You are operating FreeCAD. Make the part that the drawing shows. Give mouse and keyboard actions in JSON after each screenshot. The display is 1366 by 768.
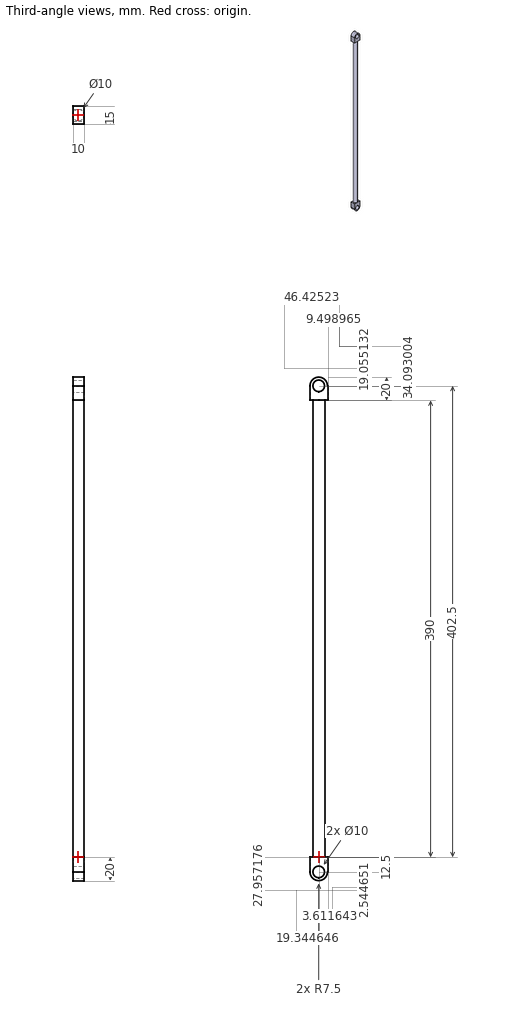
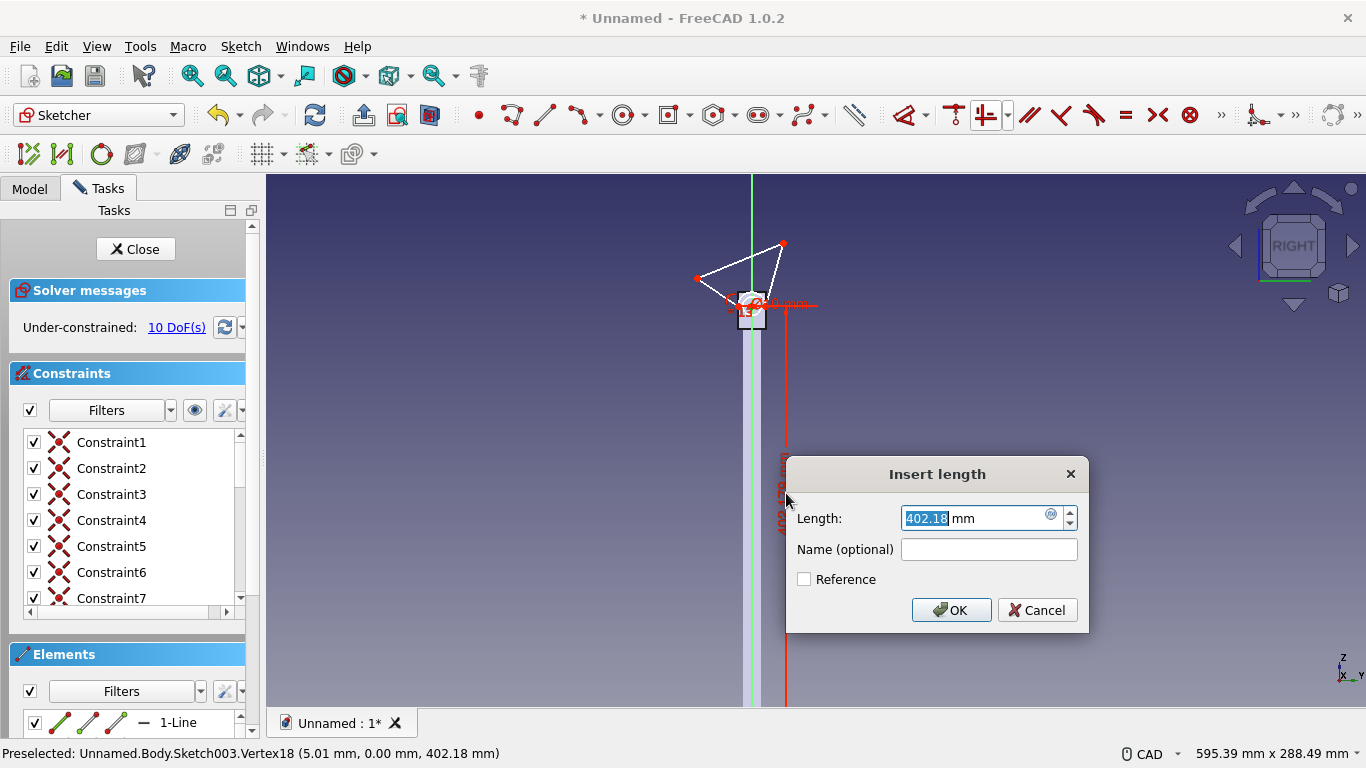
{"action": "type", "text": "402.5"}
{"action": "key", "text": "Return"}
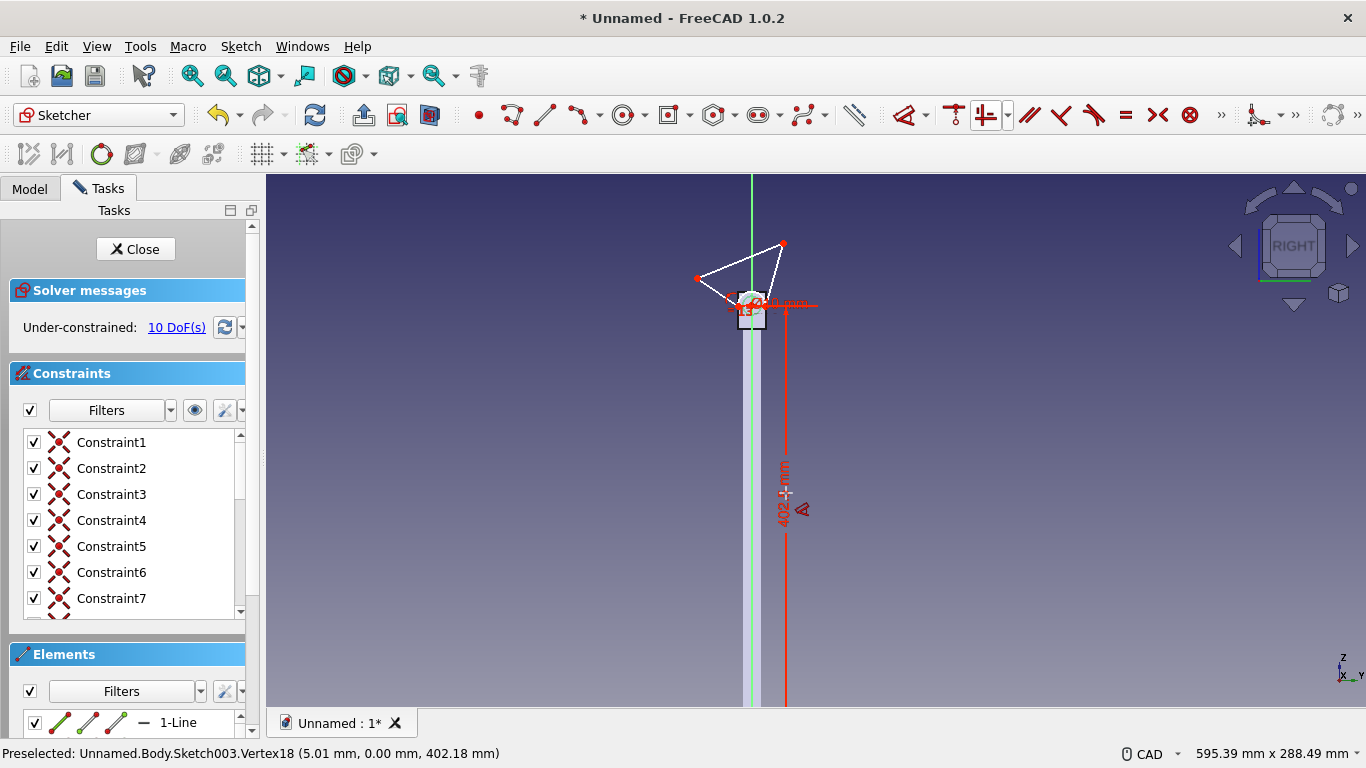
{"action": "left_click", "coordinate": [766, 306]}
{"action": "left_click", "coordinate": [800, 407]}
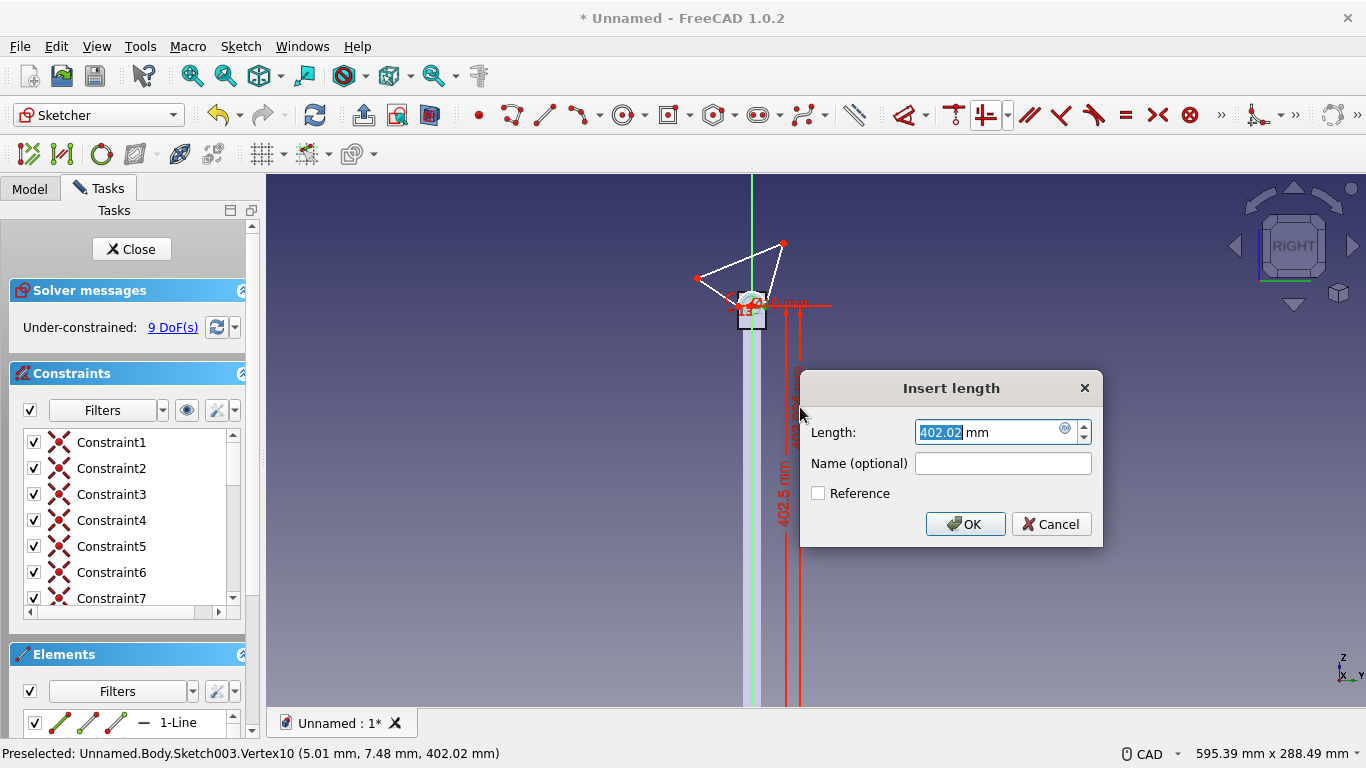
{"action": "type", "text": "402.5"}
{"action": "key", "text": "Return"}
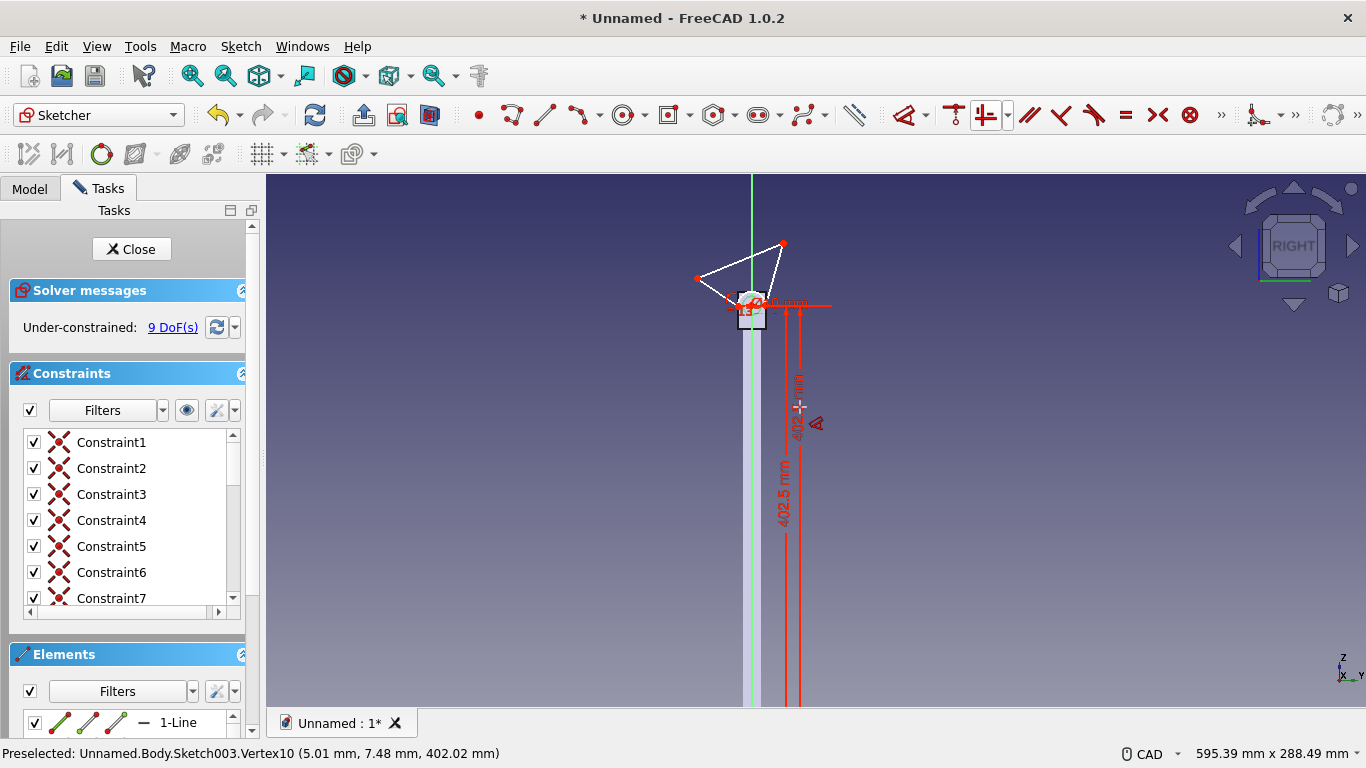
{"action": "left_click", "coordinate": [738, 306]}
{"action": "left_click", "coordinate": [786, 578]}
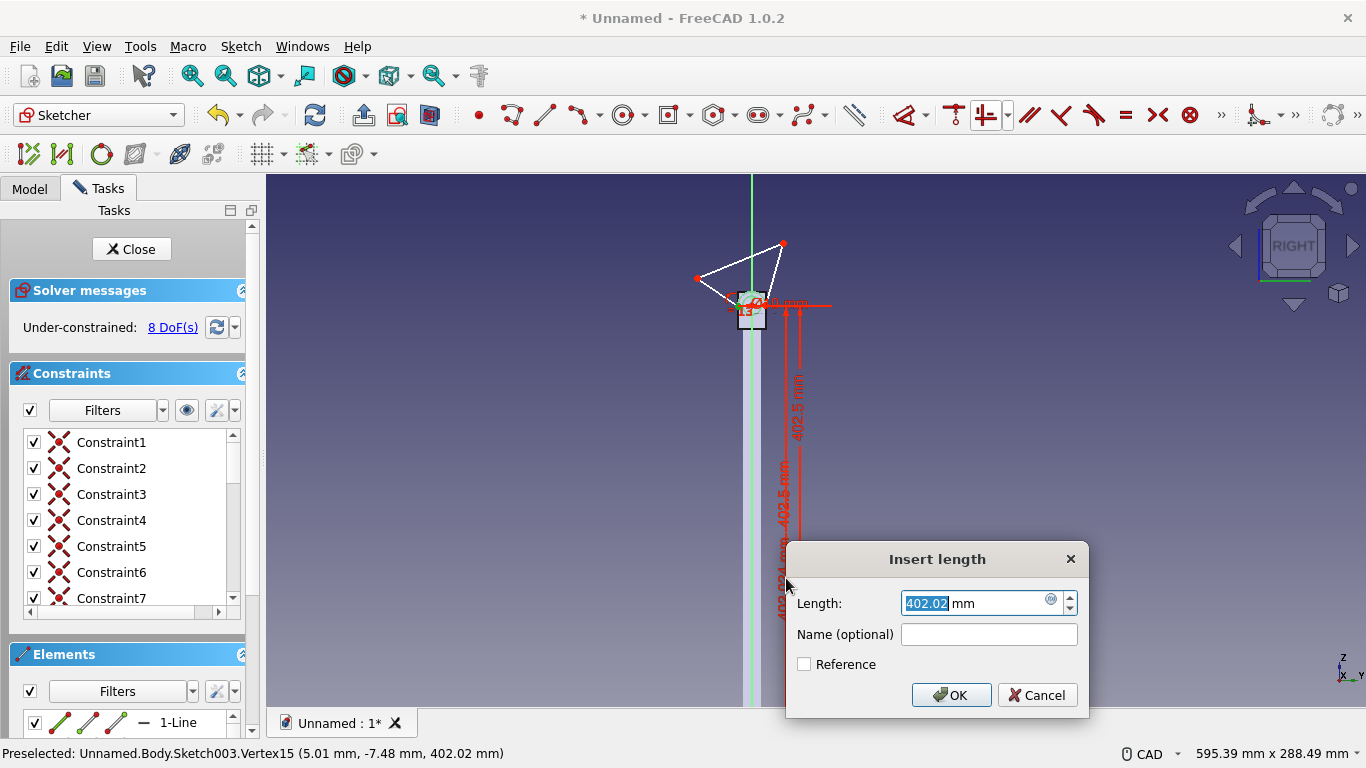
{"action": "type", "text": "402.5"}
{"action": "key", "text": "Return"}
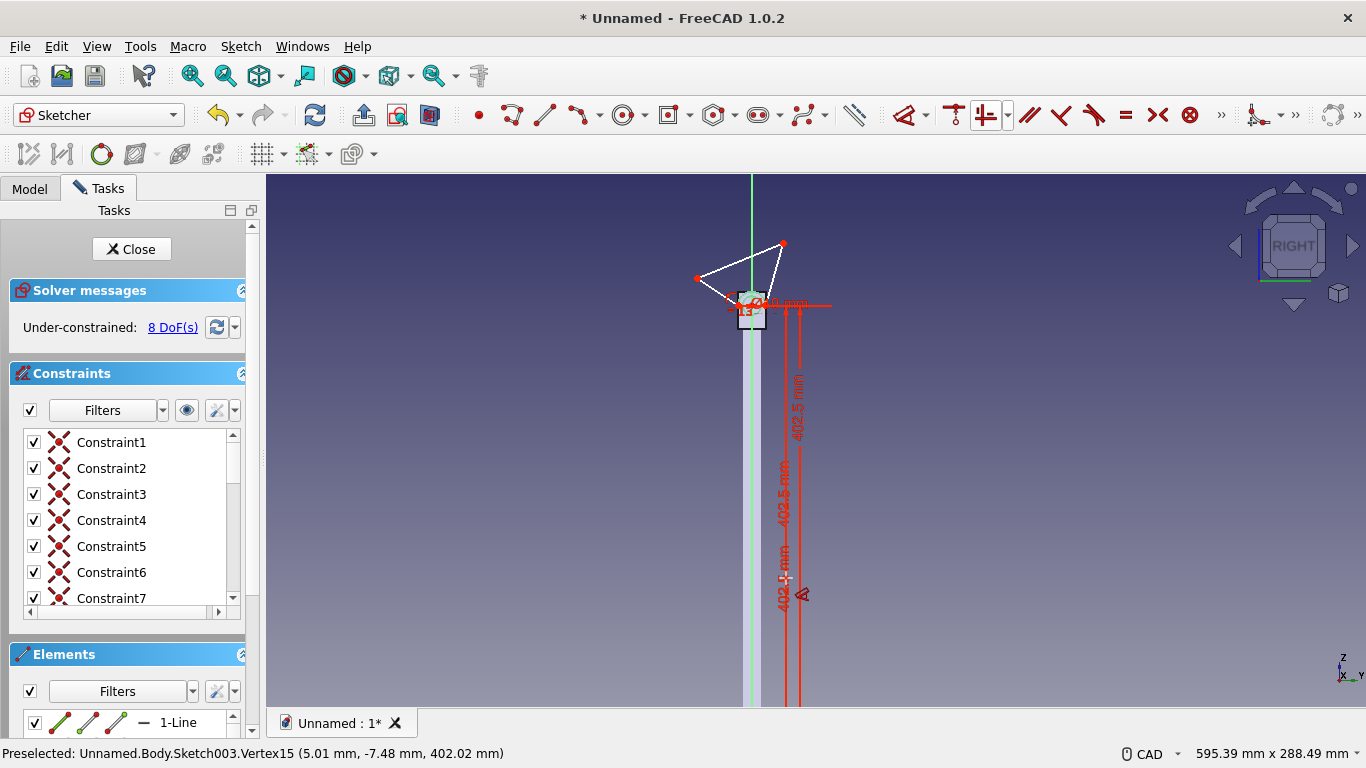
{"action": "scroll", "coordinate": [752, 306], "scroll_direction": "down", "scroll_amount": 5}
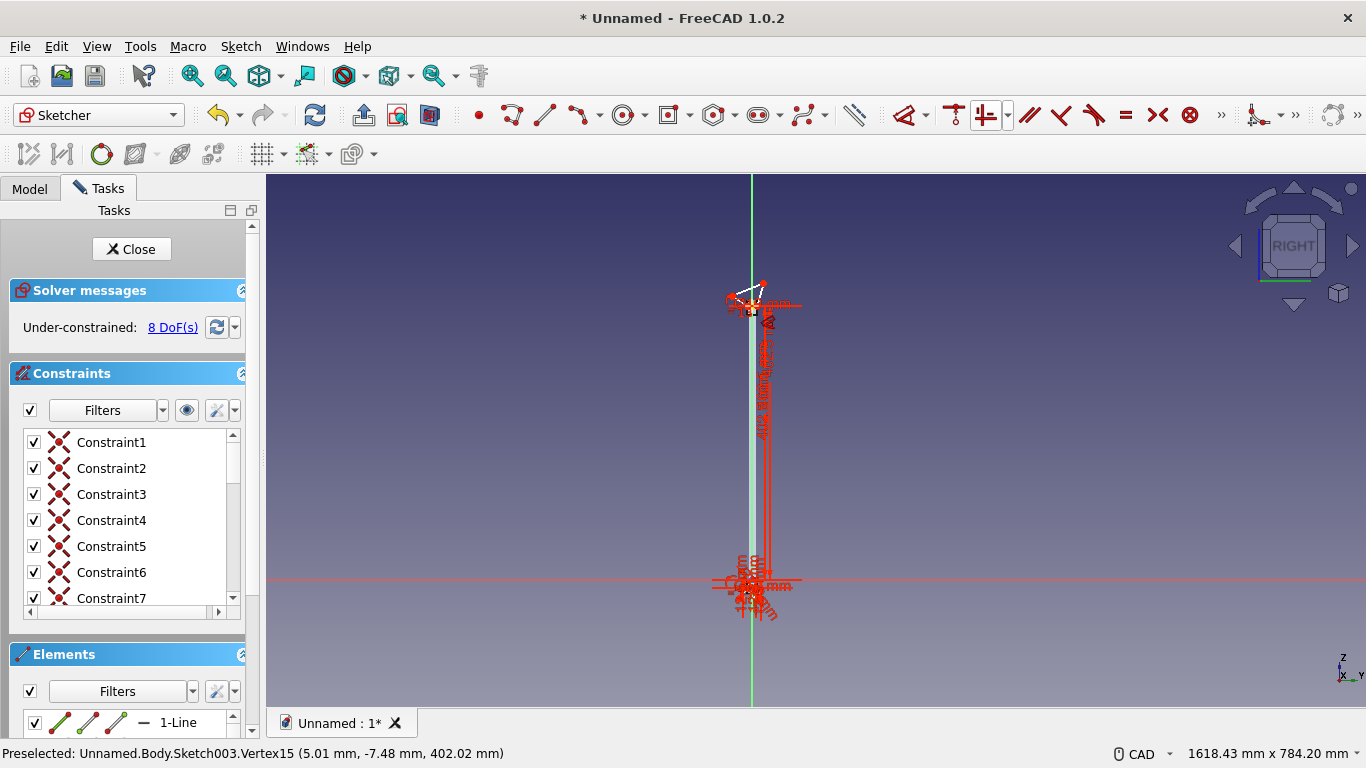
{"action": "scroll", "coordinate": [745, 598], "scroll_direction": "up", "scroll_amount": 16}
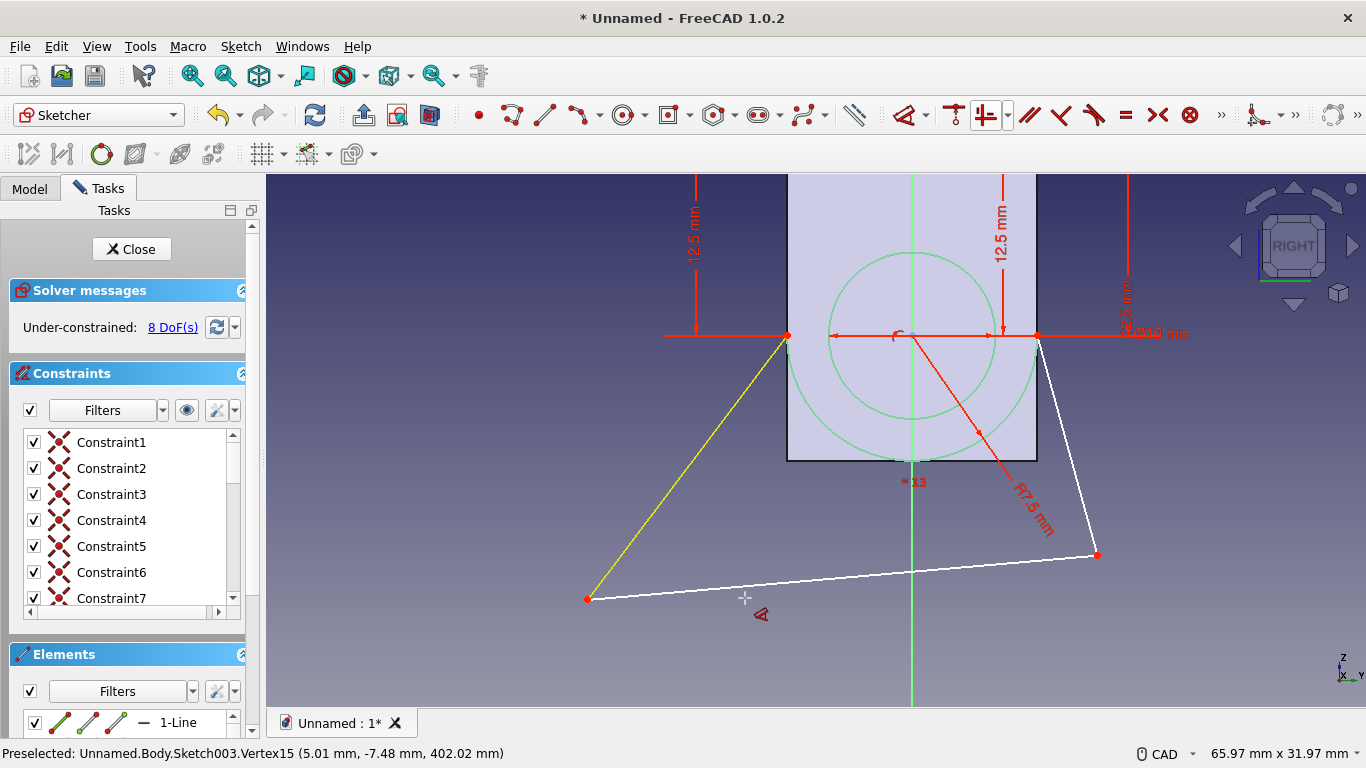
{"action": "left_click", "coordinate": [741, 587]}
{"action": "left_click", "coordinate": [1132, 578]}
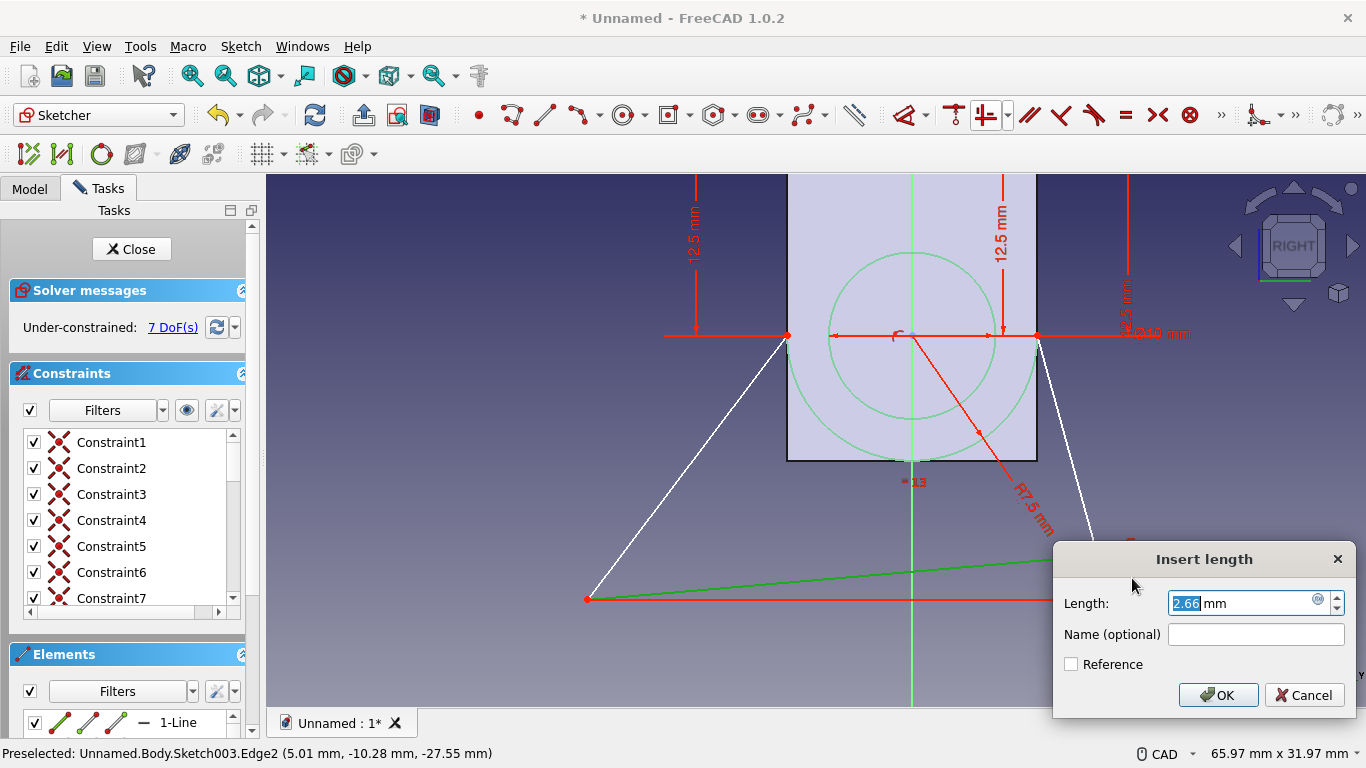
{"action": "type", "text": "2.544651"}
{"action": "key", "text": "Return"}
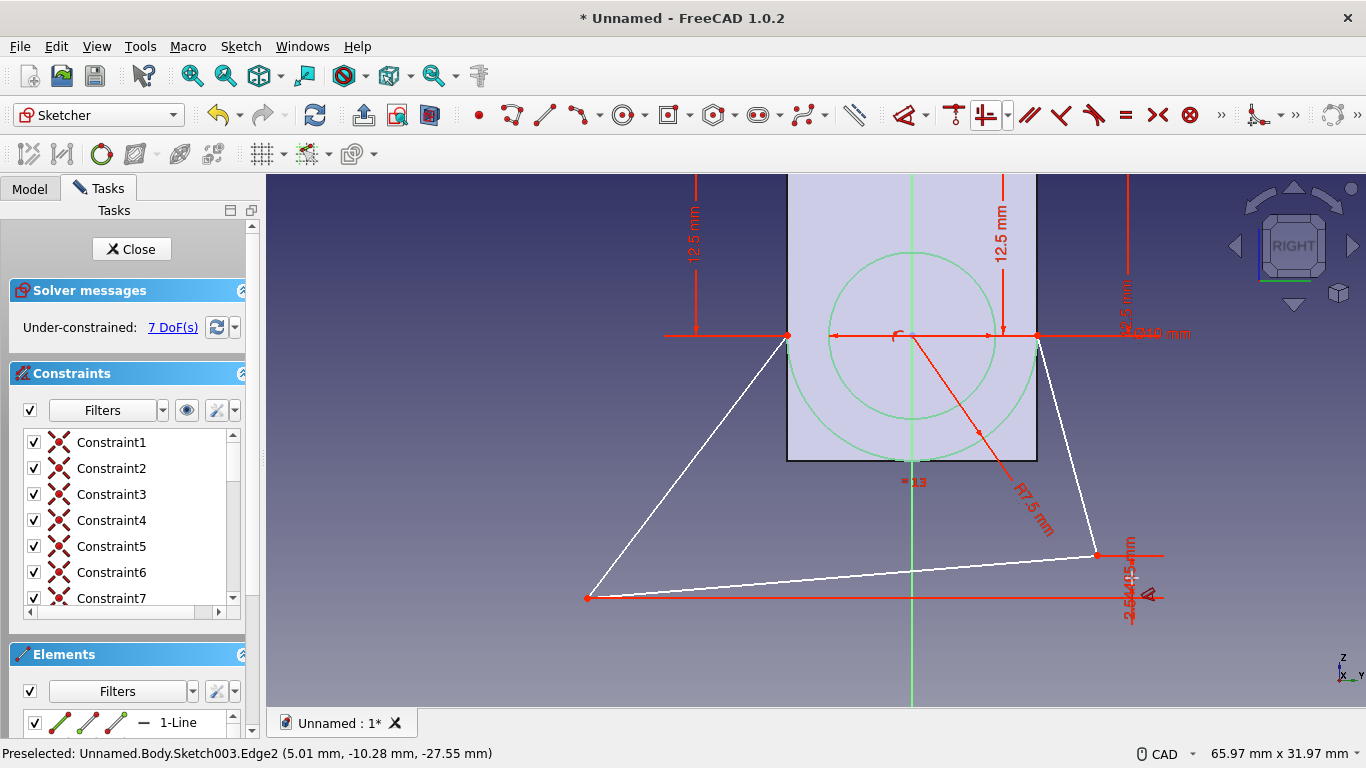
{"action": "left_click", "coordinate": [1080, 490]}
{"action": "left_click", "coordinate": [1054, 590]}